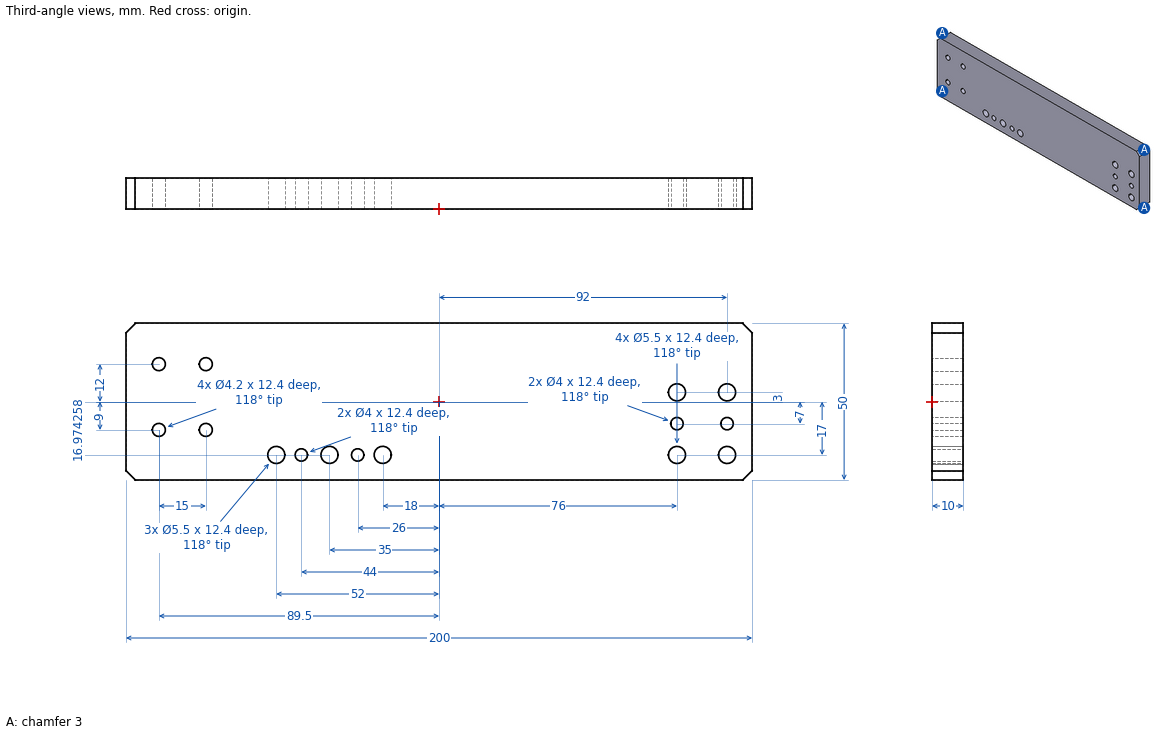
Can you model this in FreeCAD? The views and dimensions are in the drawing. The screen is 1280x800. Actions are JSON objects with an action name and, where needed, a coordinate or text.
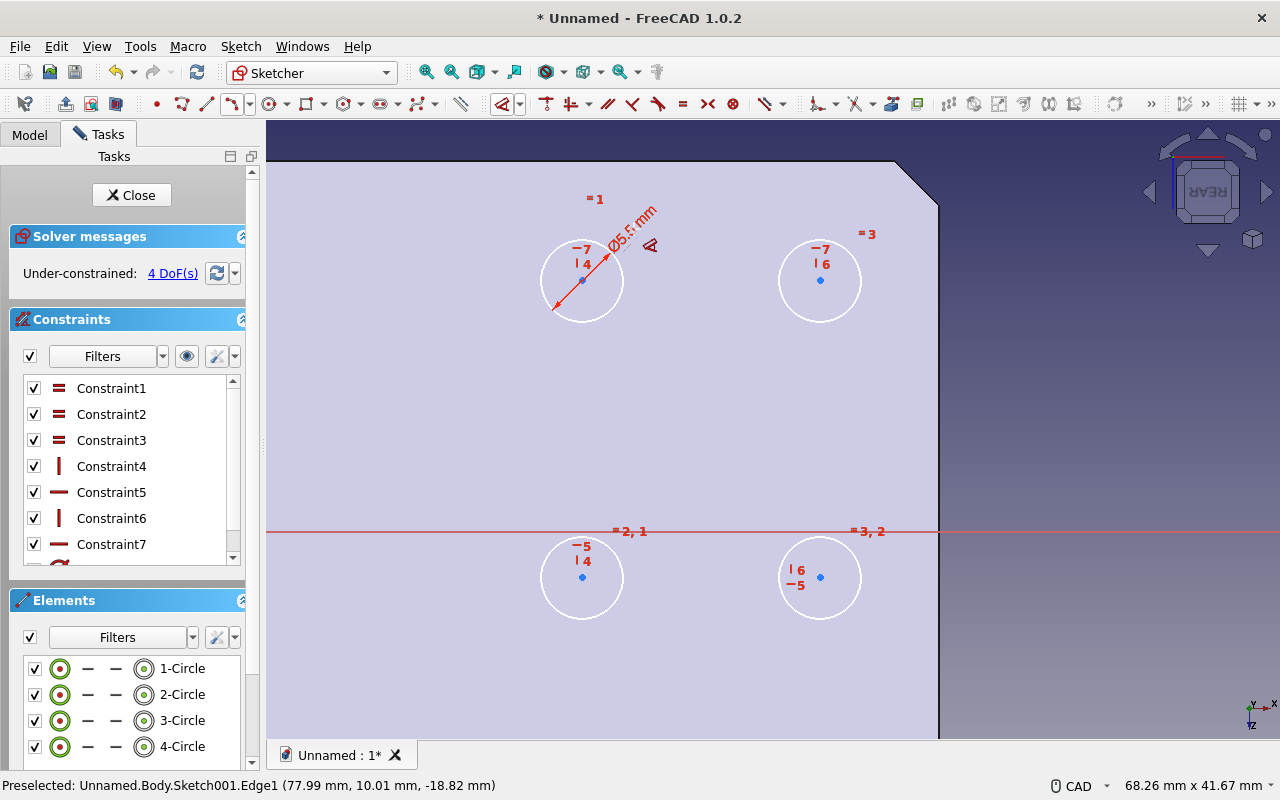
{"action": "left_click", "coordinate": [582, 578]}
{"action": "left_click", "coordinate": [640, 555]}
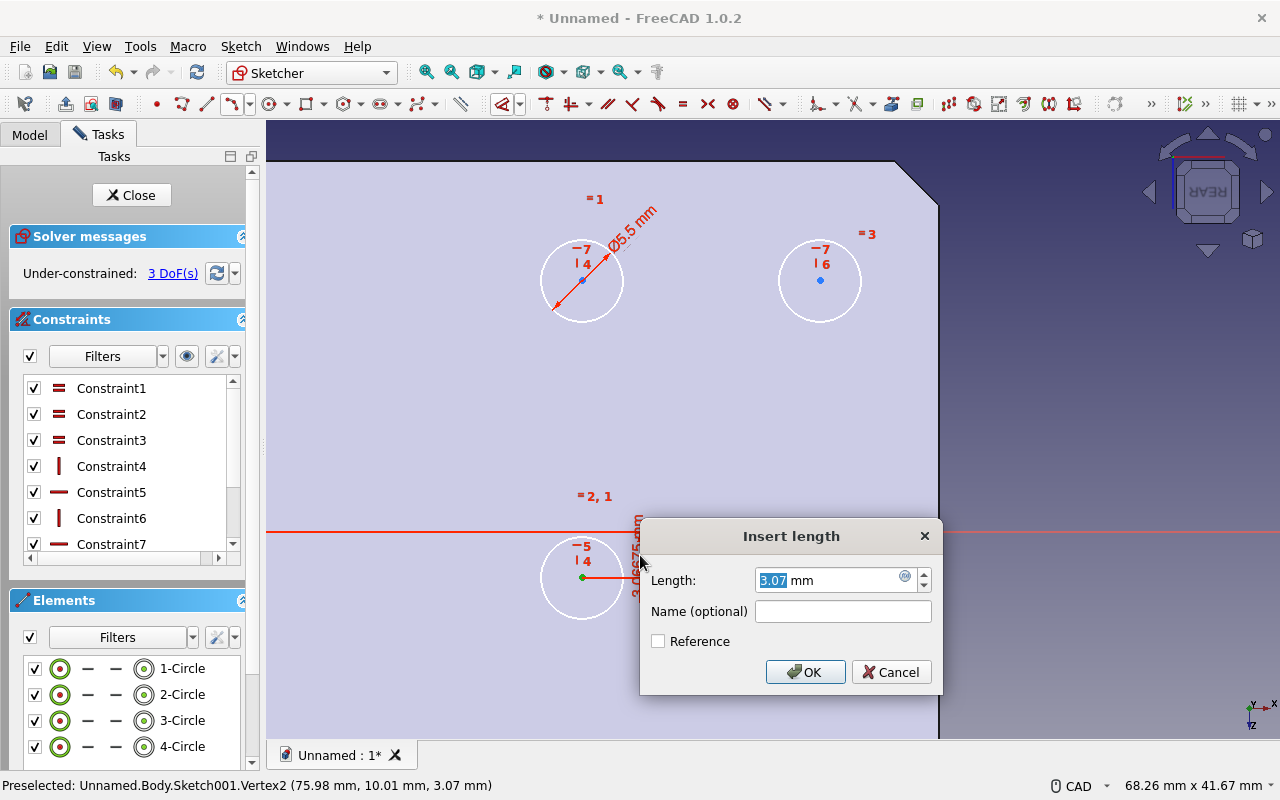
{"action": "type", "text": "3"}
{"action": "key", "text": "Return"}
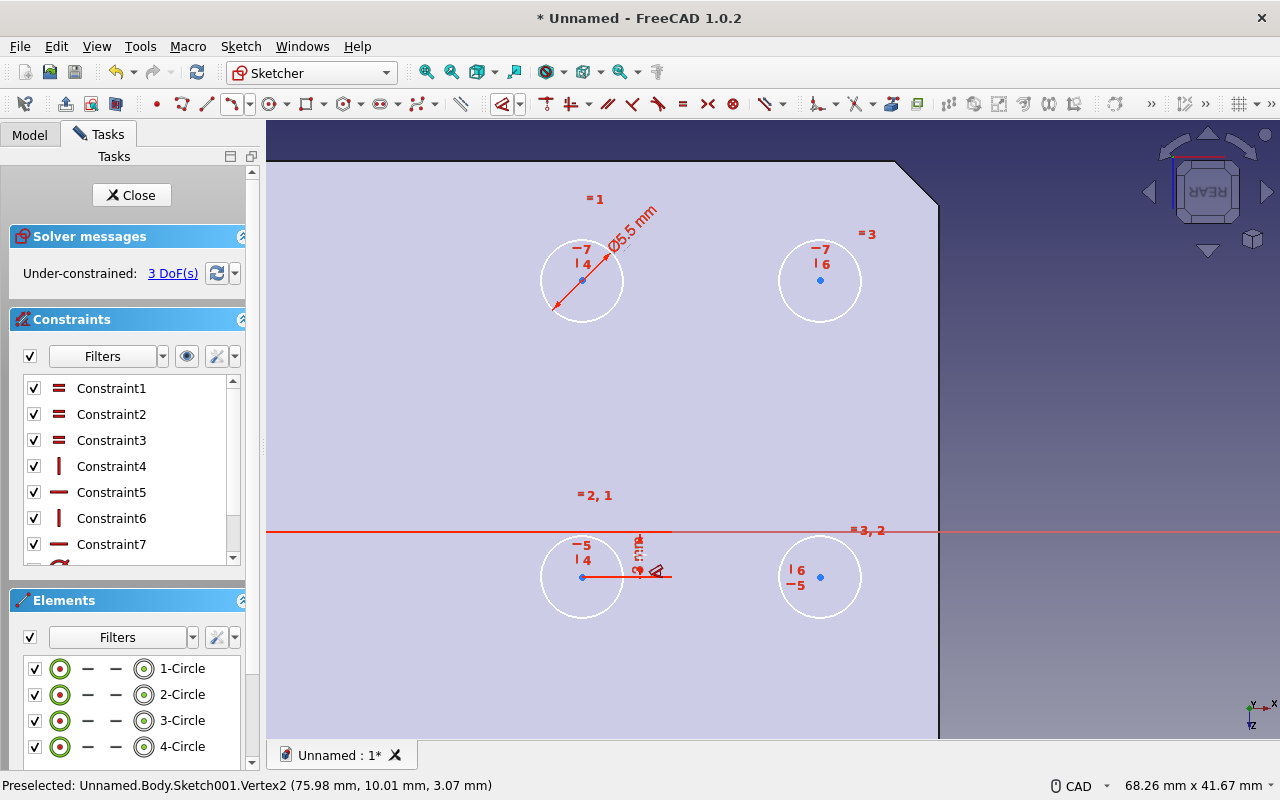
{"action": "left_click", "coordinate": [582, 281]}
{"action": "left_click", "coordinate": [438, 247]}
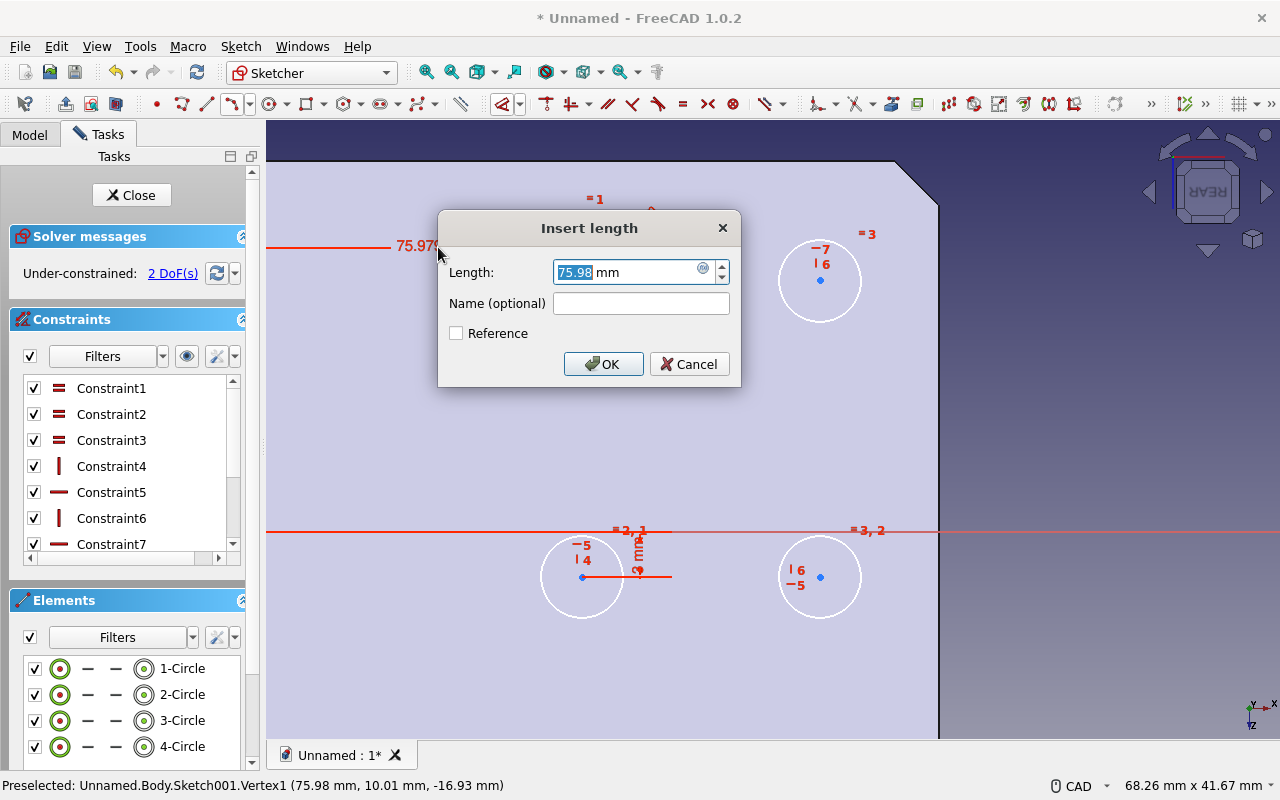
{"action": "type", "text": "76"}
{"action": "key", "text": "Return"}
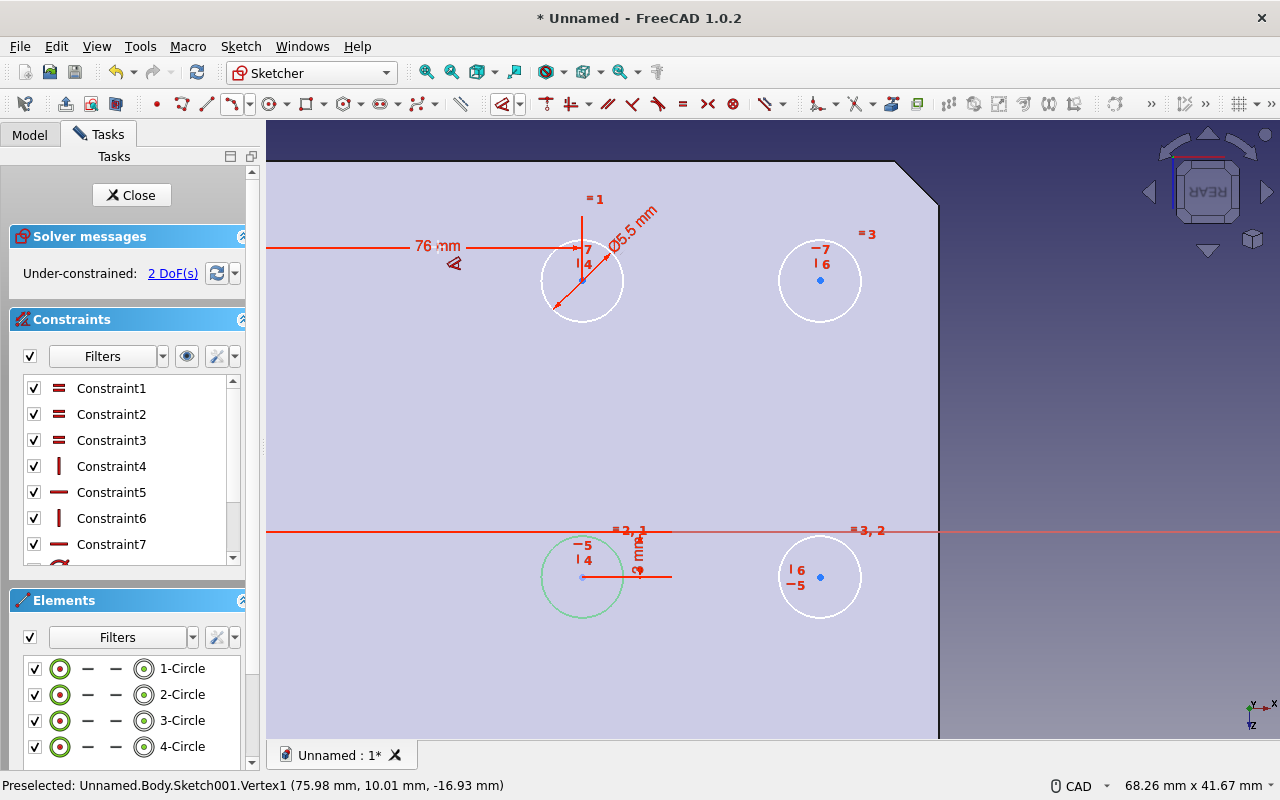
{"action": "left_click", "coordinate": [582, 281]}
{"action": "left_click", "coordinate": [616, 407]}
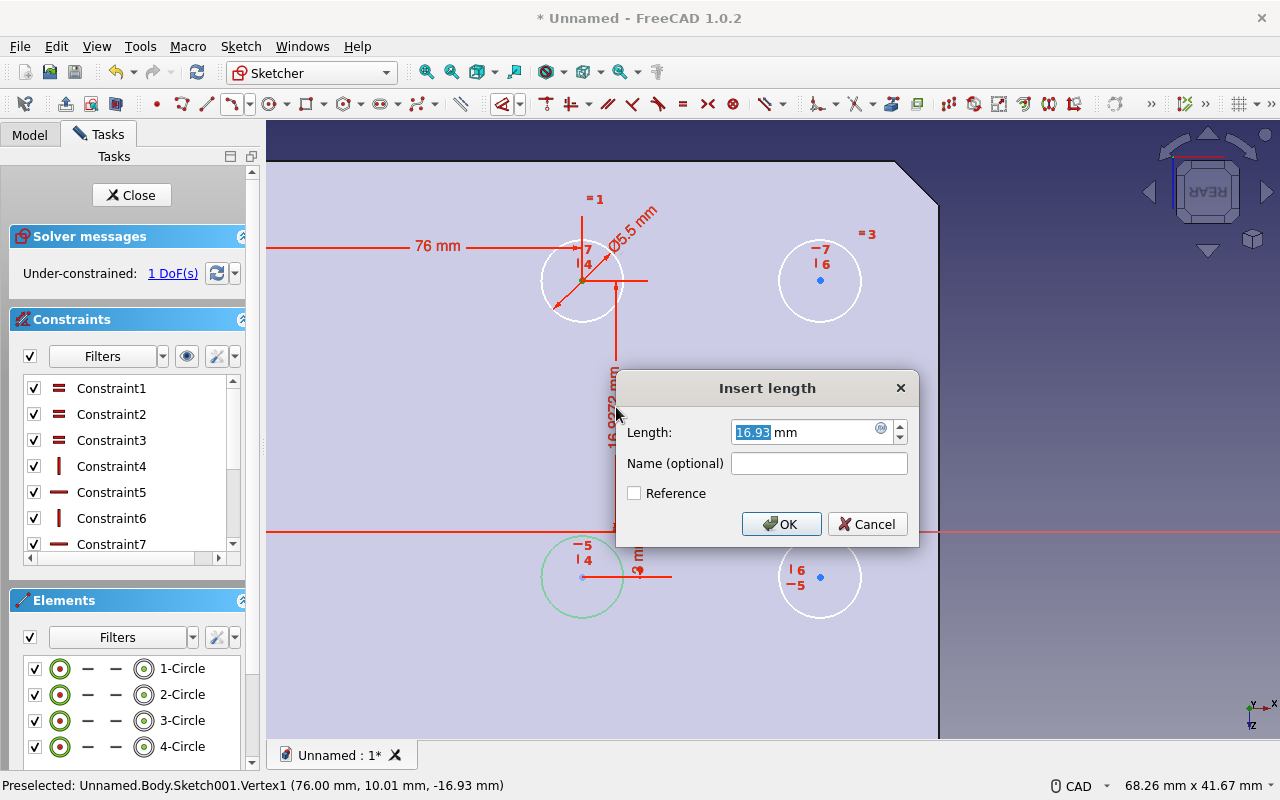
{"action": "type", "text": "17"}
{"action": "key", "text": "Return"}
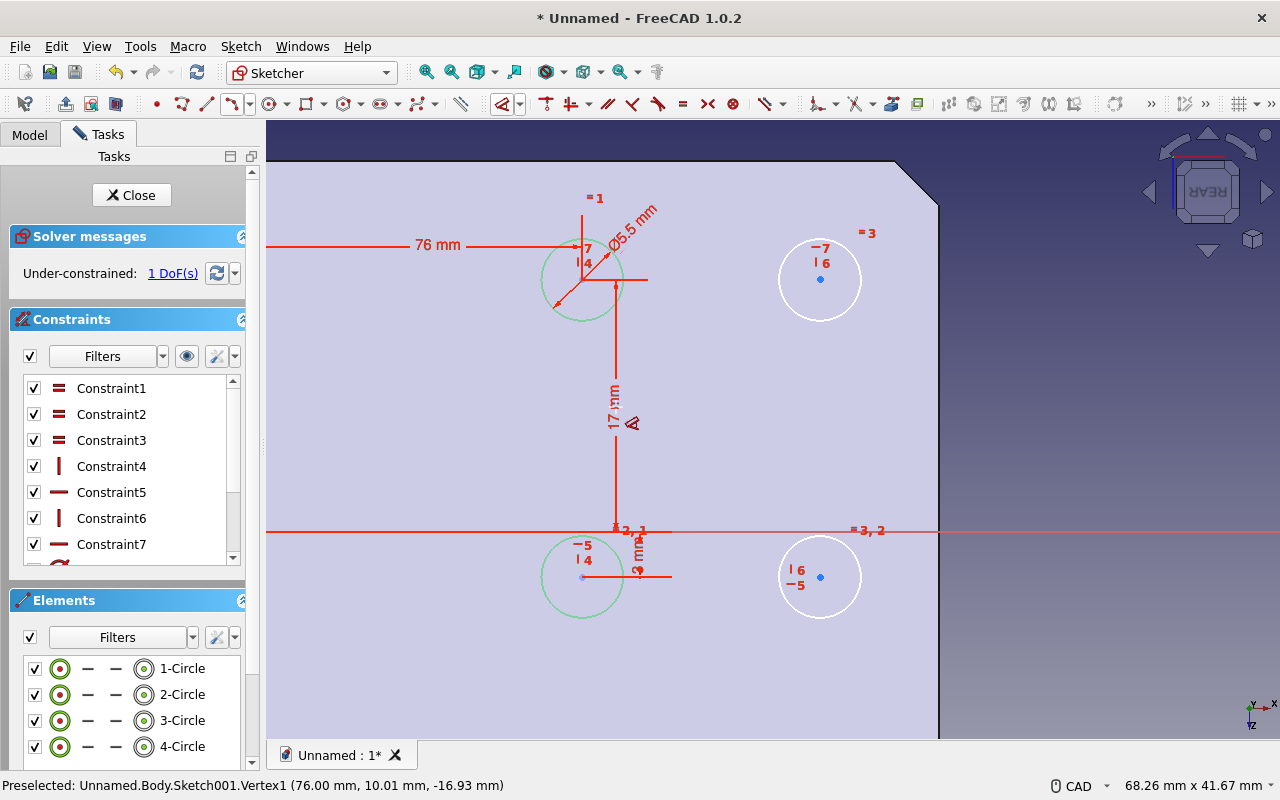
{"action": "left_click", "coordinate": [820, 577]}
{"action": "left_click", "coordinate": [436, 611]}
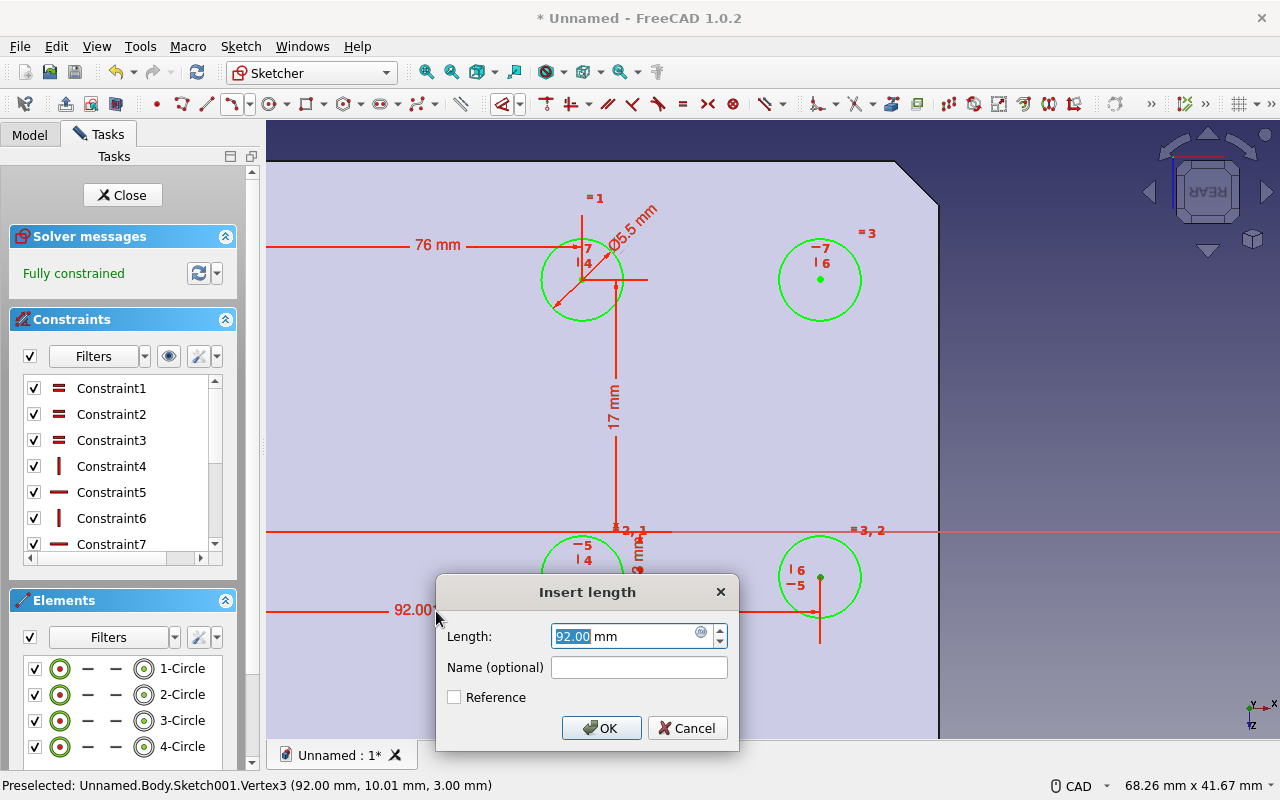
{"action": "type", "text": "92"}
{"action": "key", "text": "Return"}
{"action": "key", "text": "Escape"}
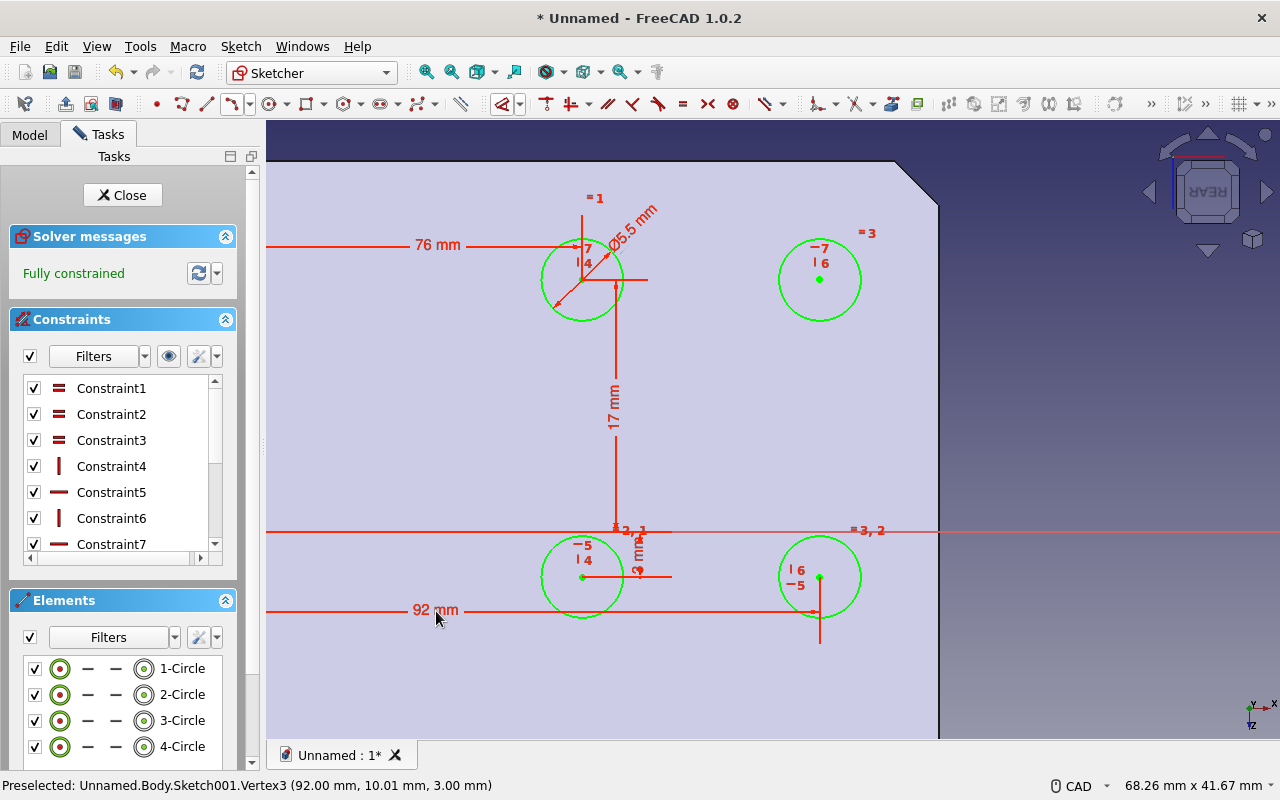
{"action": "left_click", "coordinate": [123, 195]}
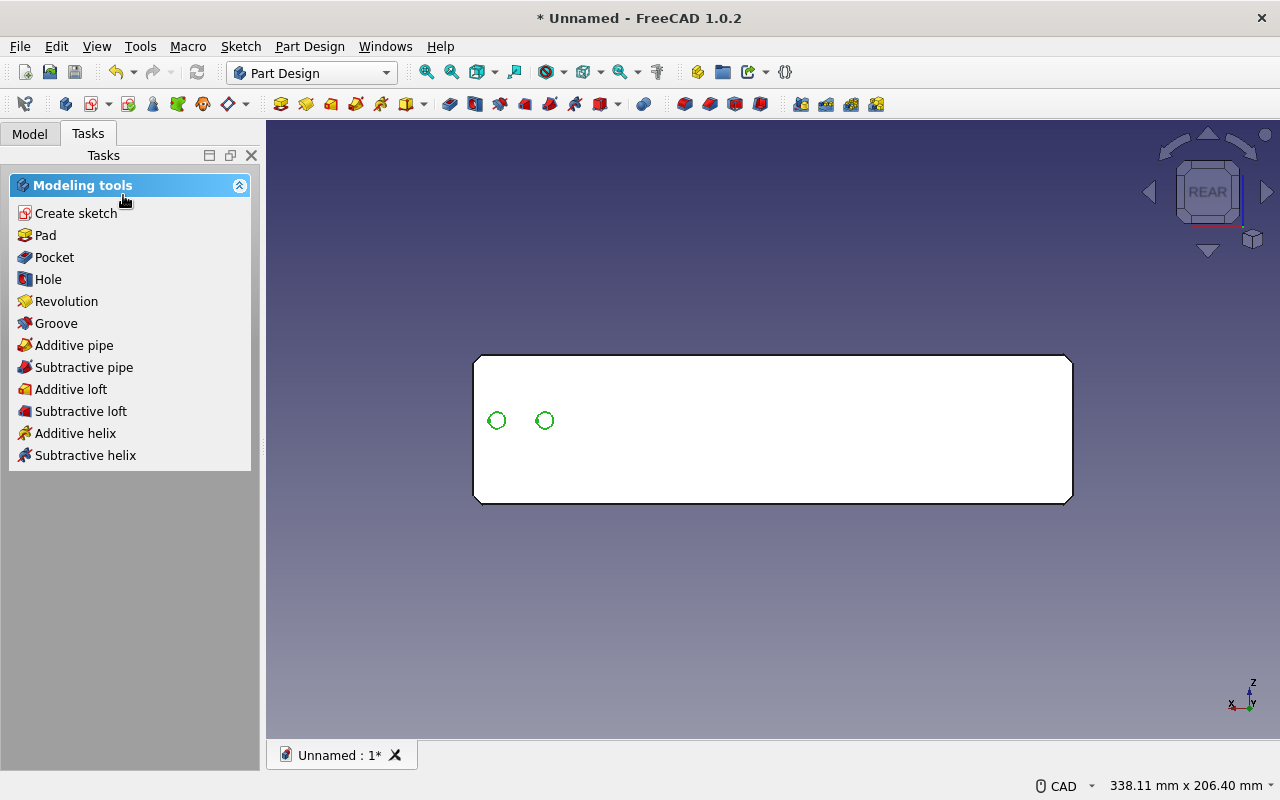
{"action": "left_click", "coordinate": [475, 104]}